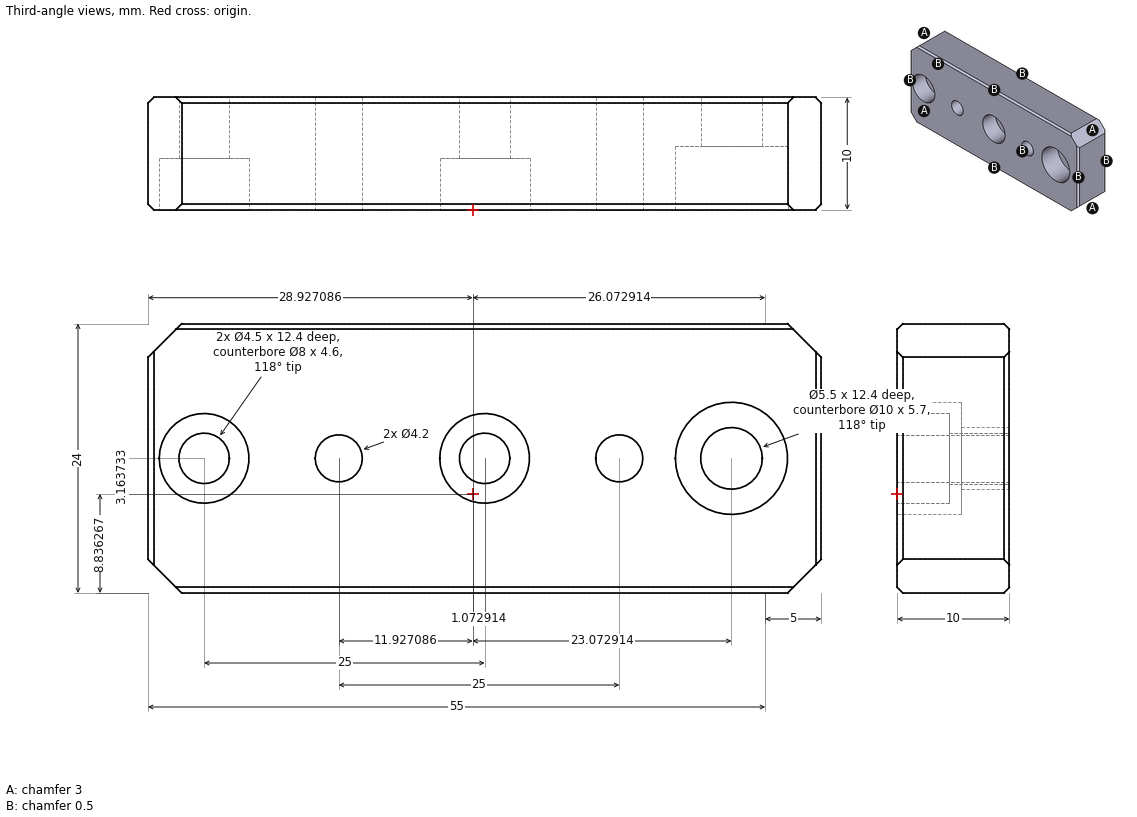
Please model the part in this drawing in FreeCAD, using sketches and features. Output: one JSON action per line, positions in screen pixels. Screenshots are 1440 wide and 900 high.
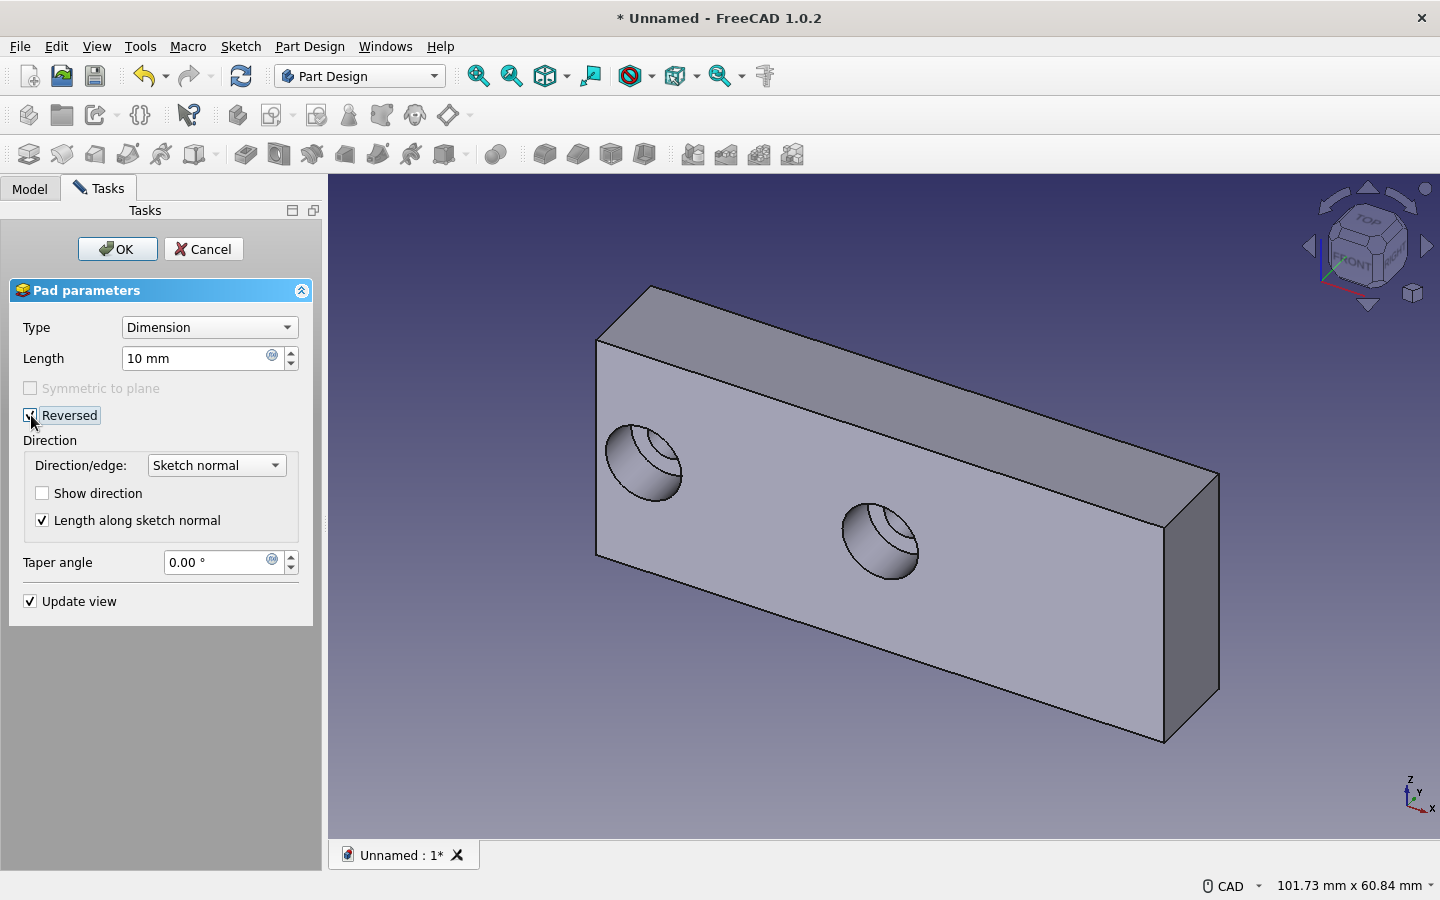
{"action": "left_click", "coordinate": [118, 249]}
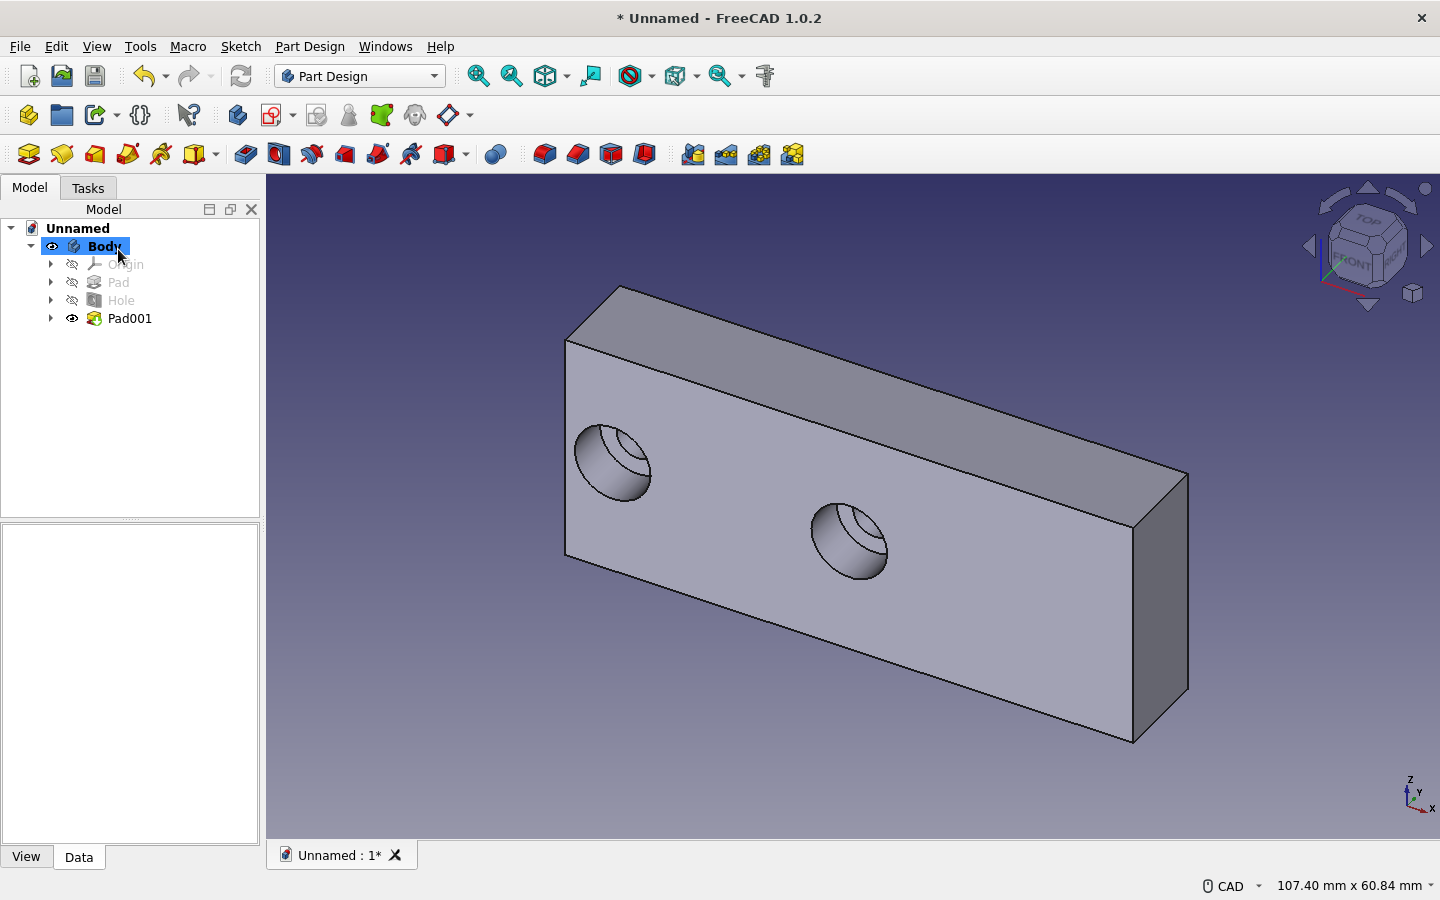
{"action": "left_click", "coordinate": [1161, 500]}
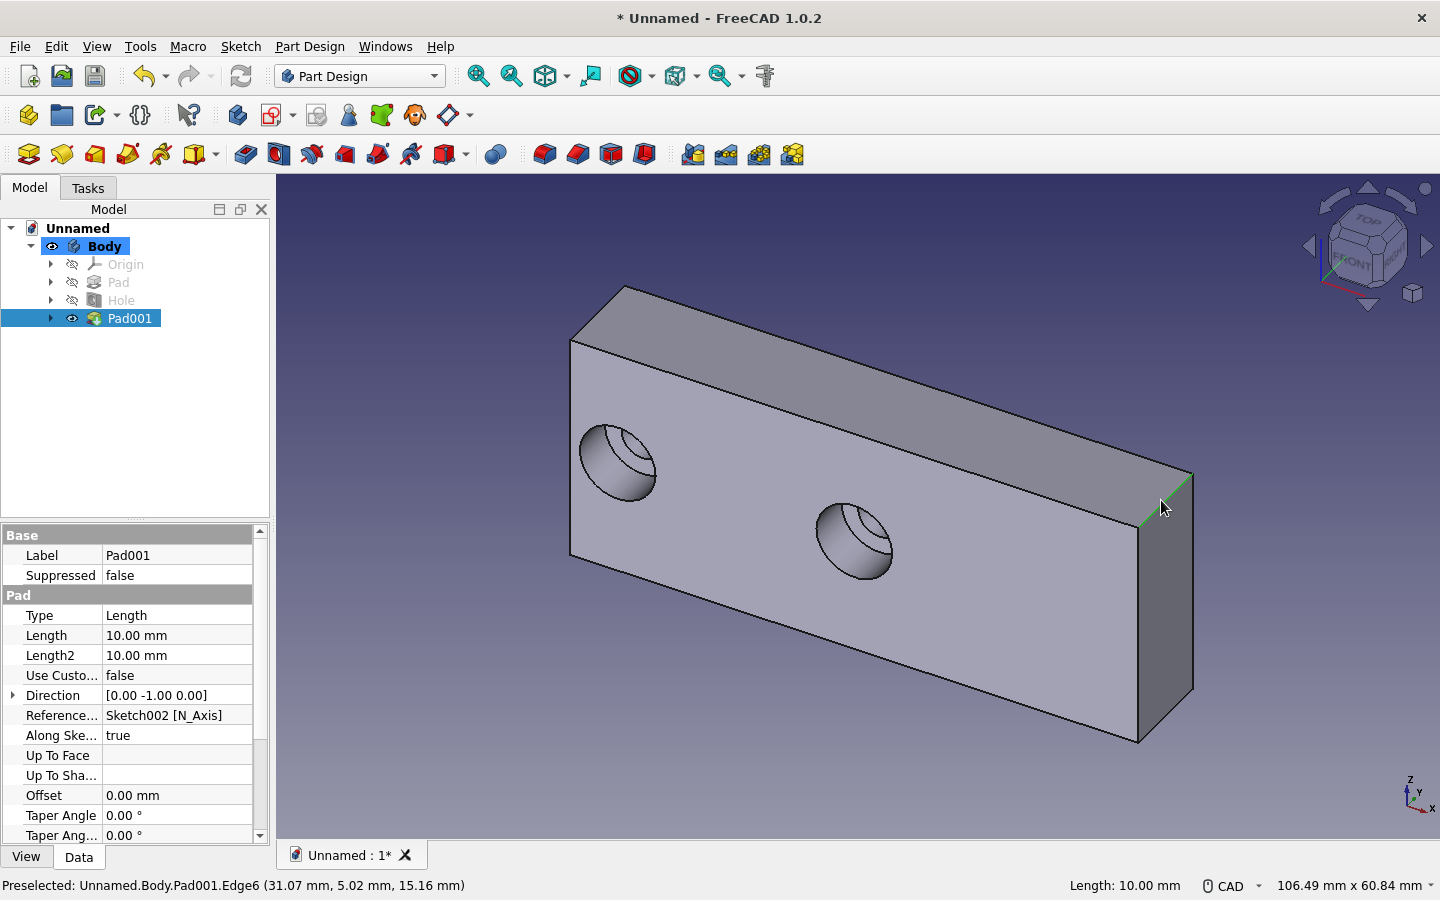
{"action": "key", "text": "0"}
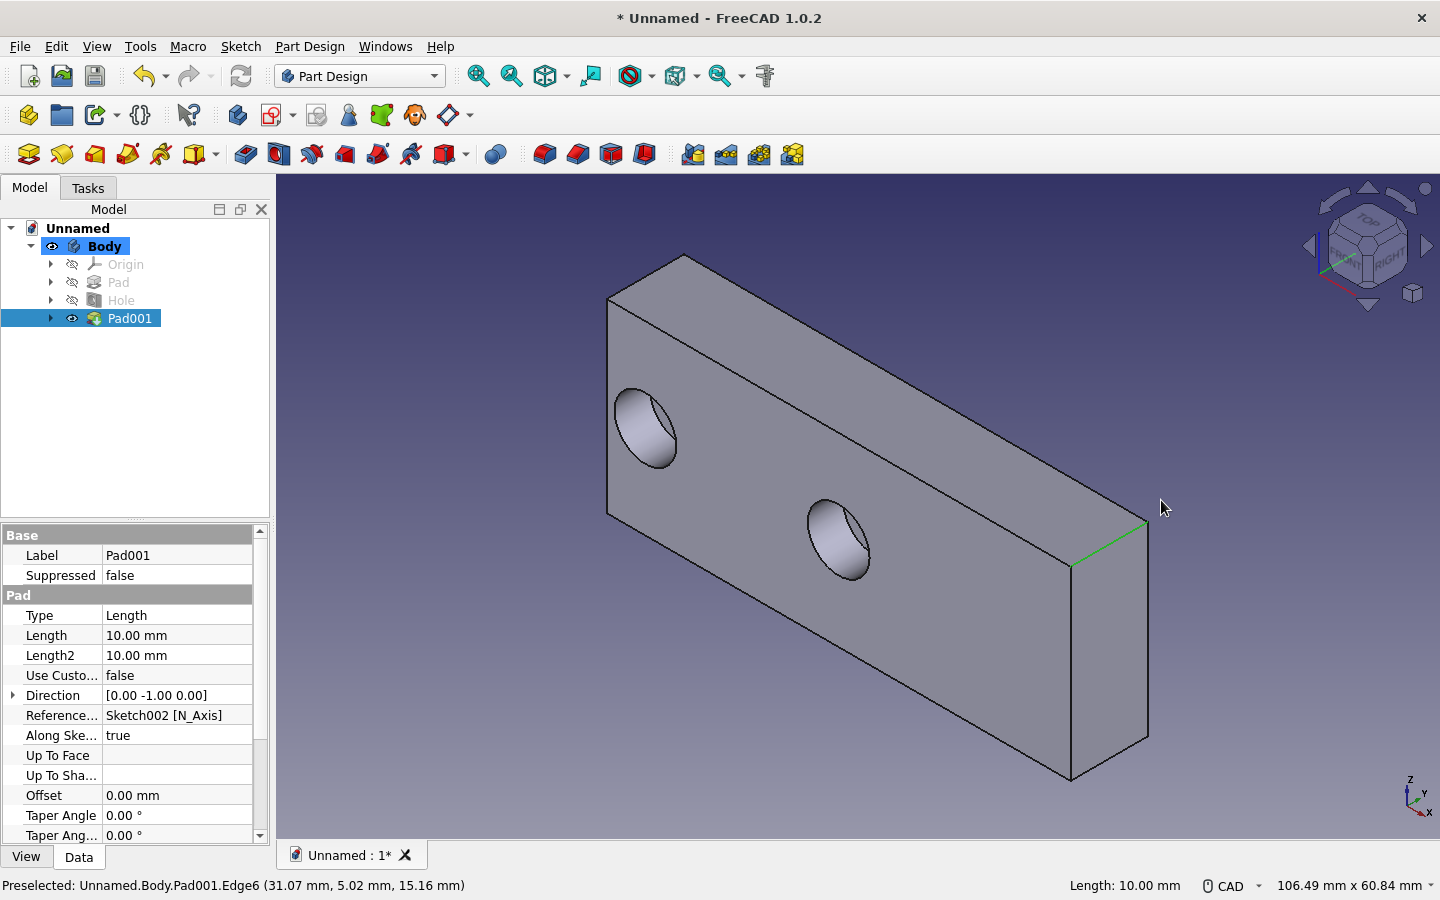
{"action": "key", "text": "2"}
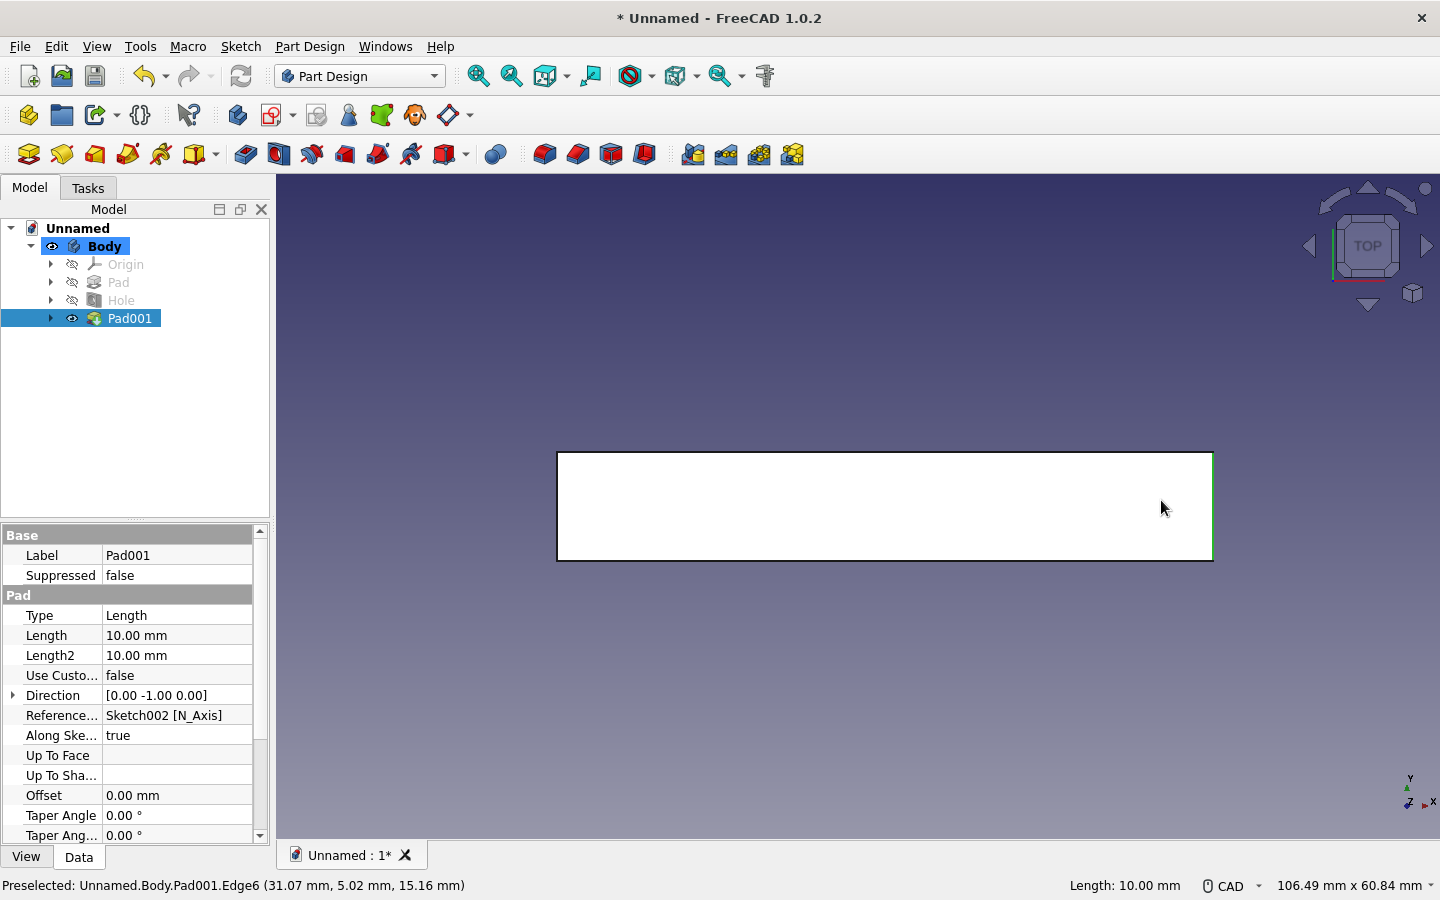
{"action": "left_click", "coordinate": [557, 505], "text": "ctrl"}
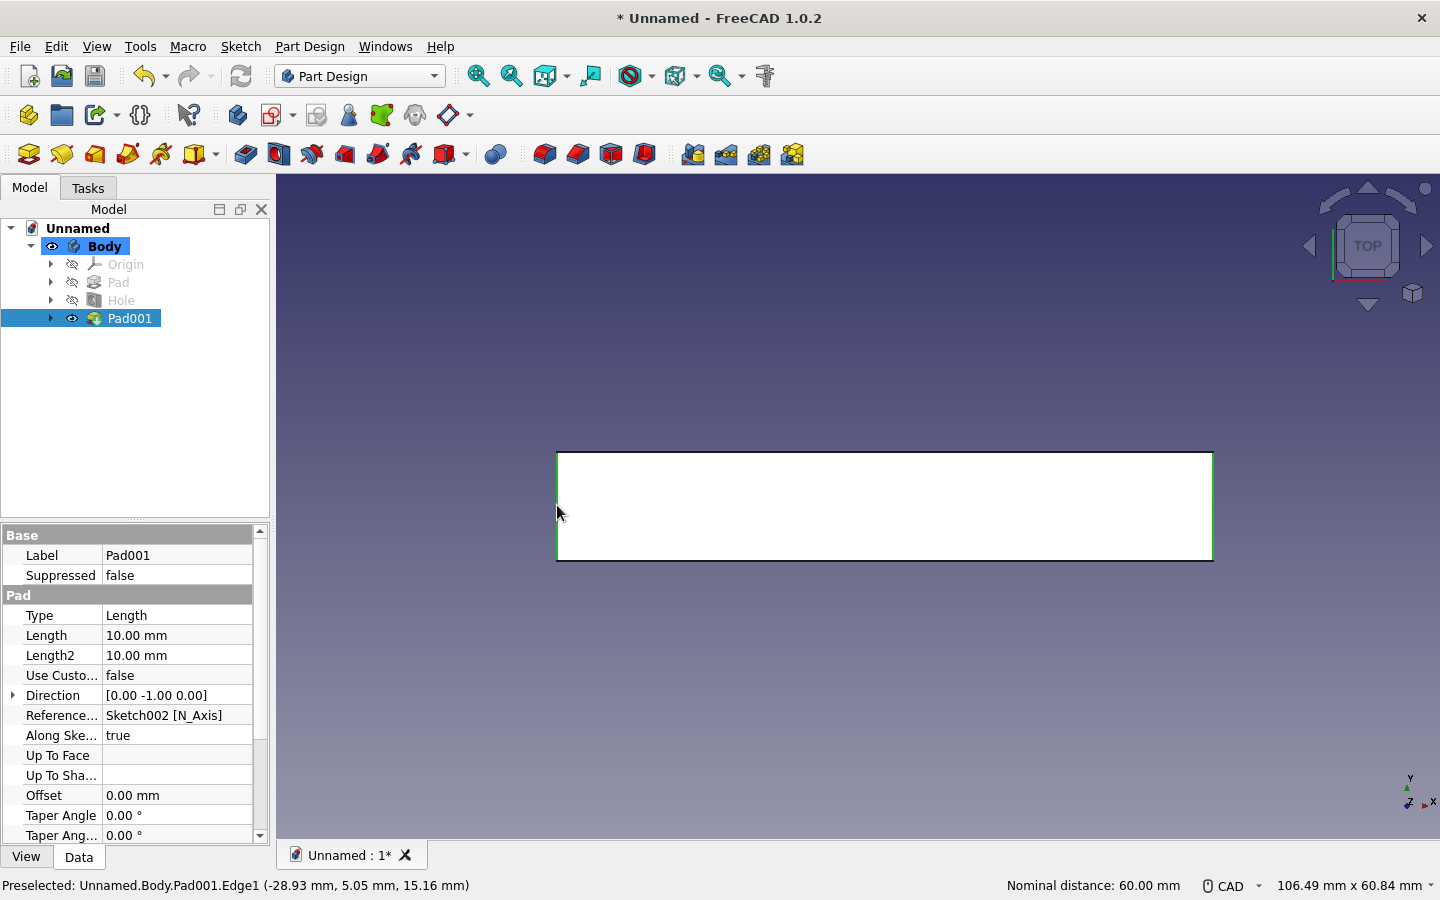
{"action": "key", "text": "1"}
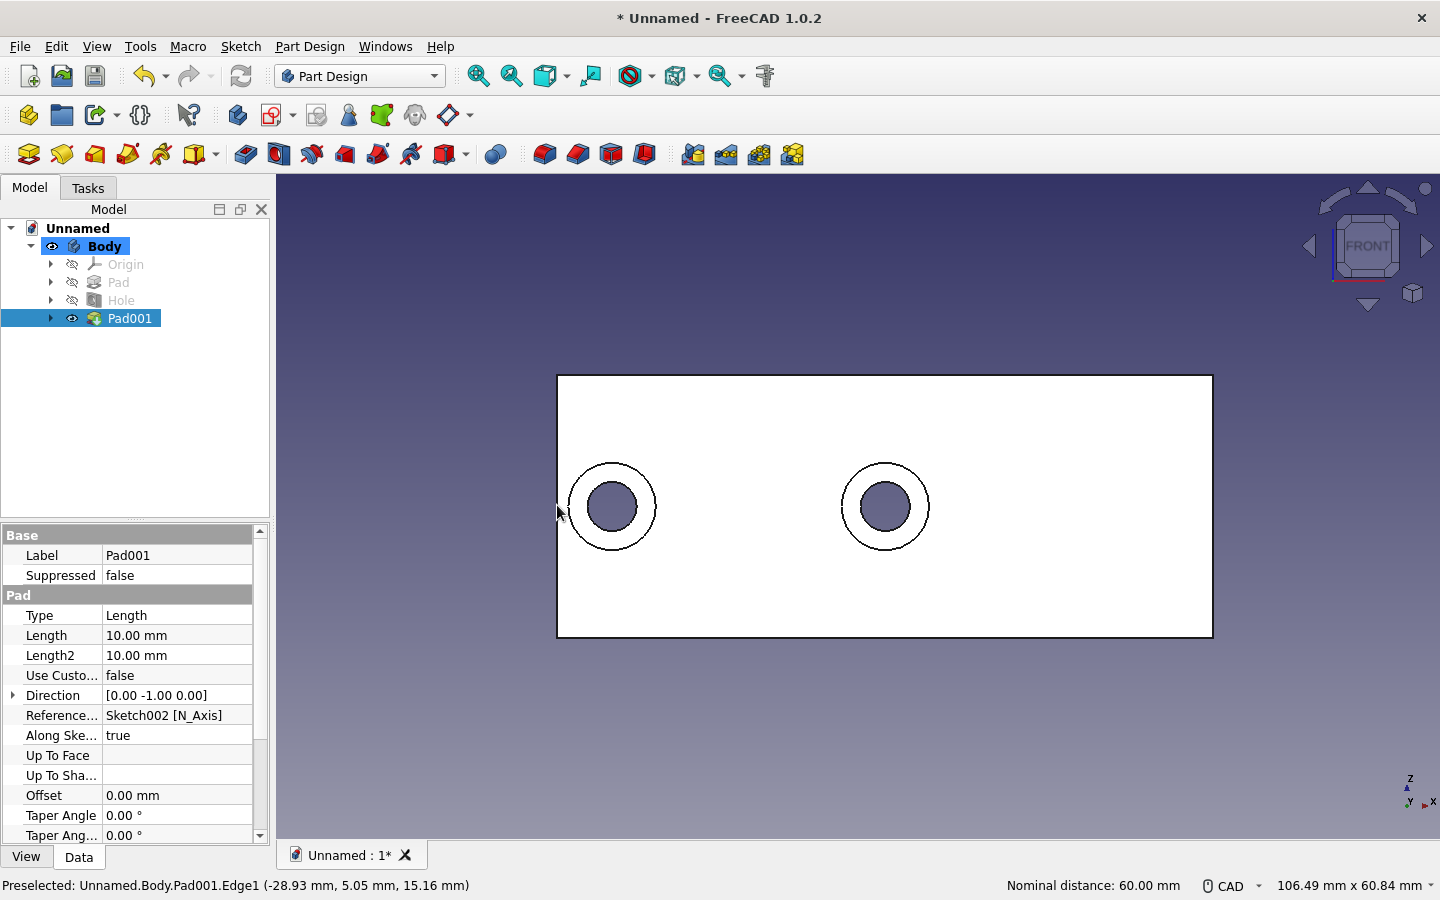
{"action": "key", "text": "3"}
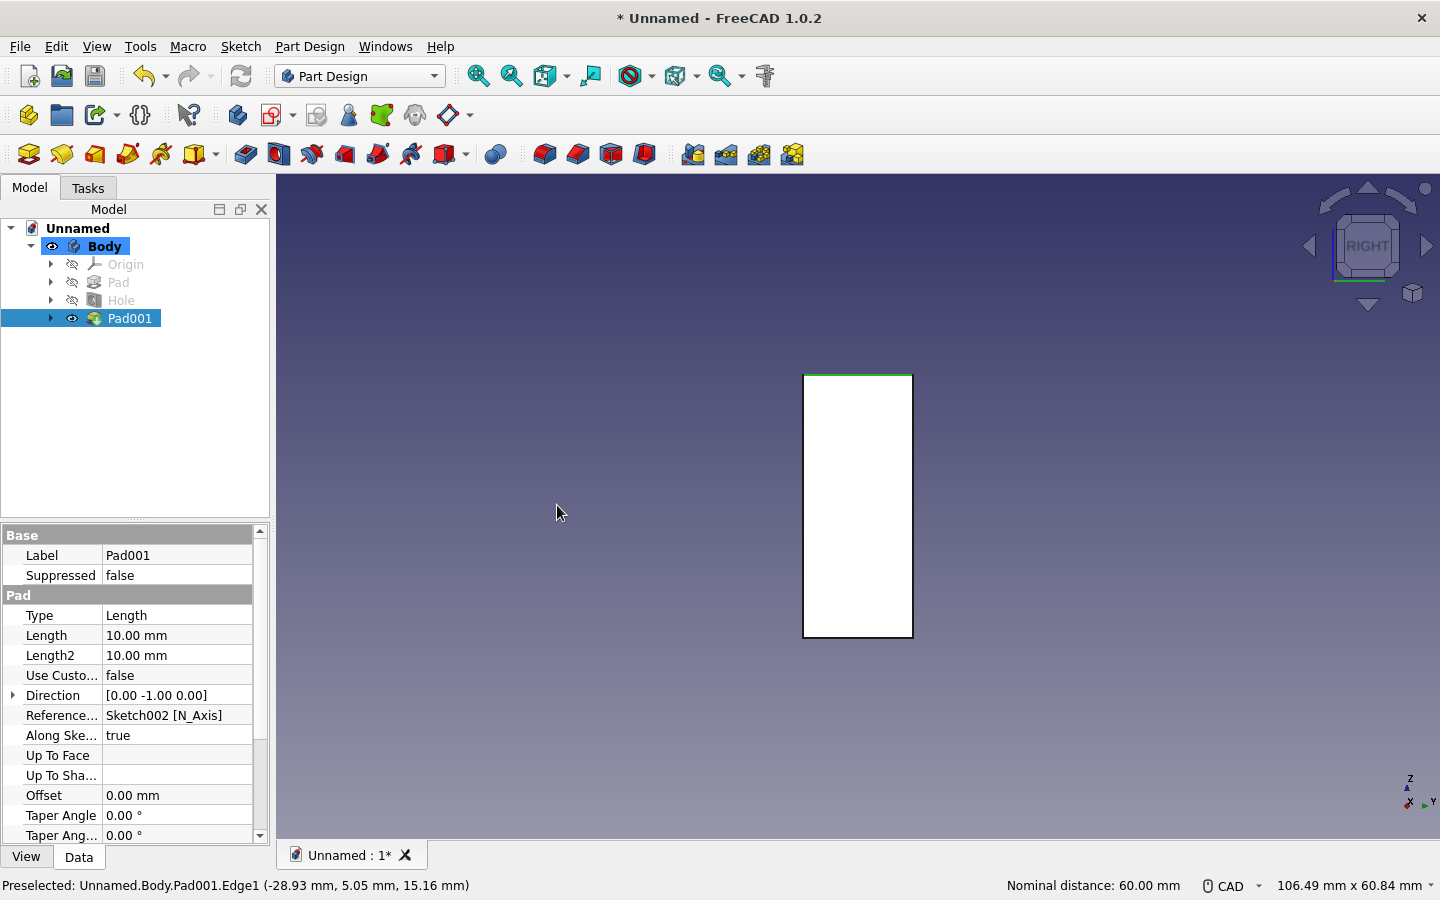
{"action": "key", "text": "v f"}